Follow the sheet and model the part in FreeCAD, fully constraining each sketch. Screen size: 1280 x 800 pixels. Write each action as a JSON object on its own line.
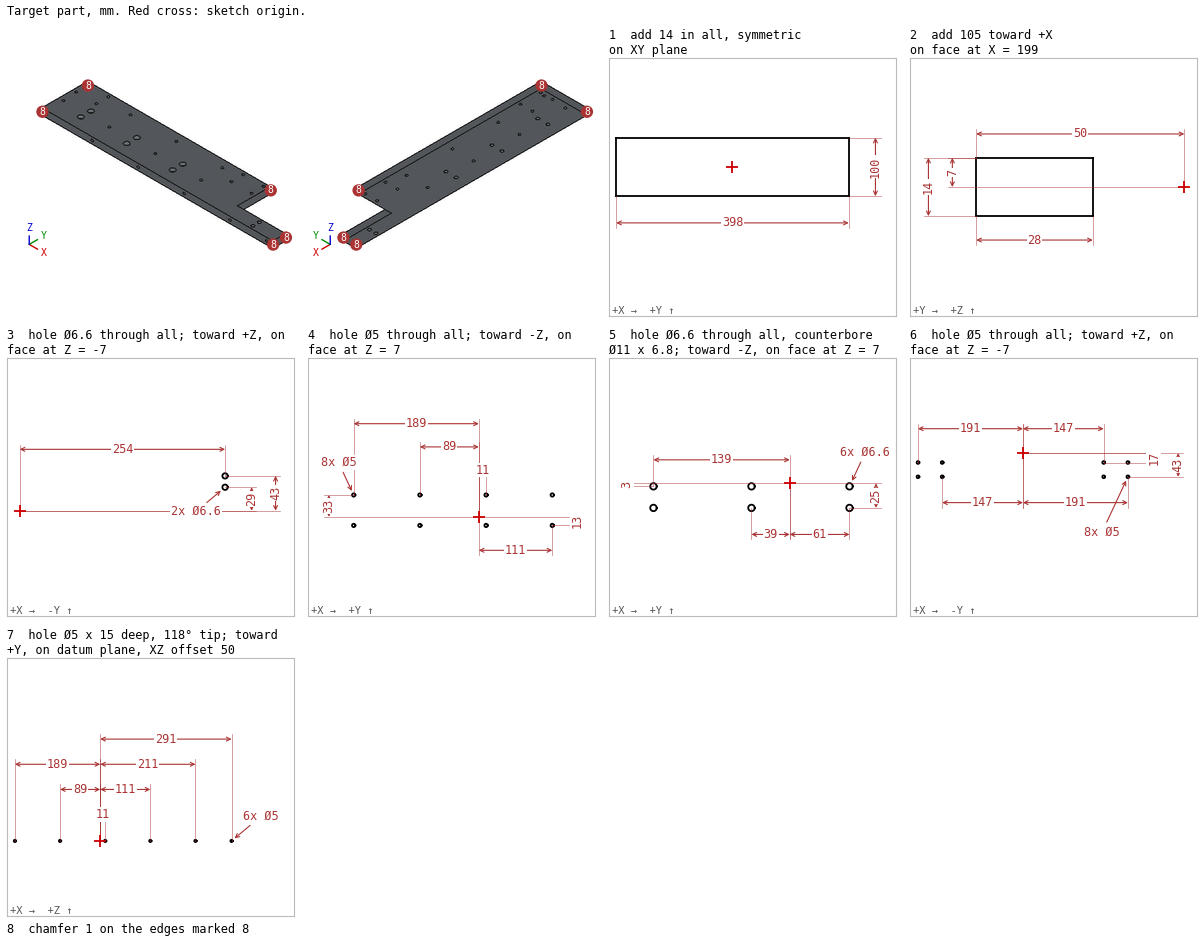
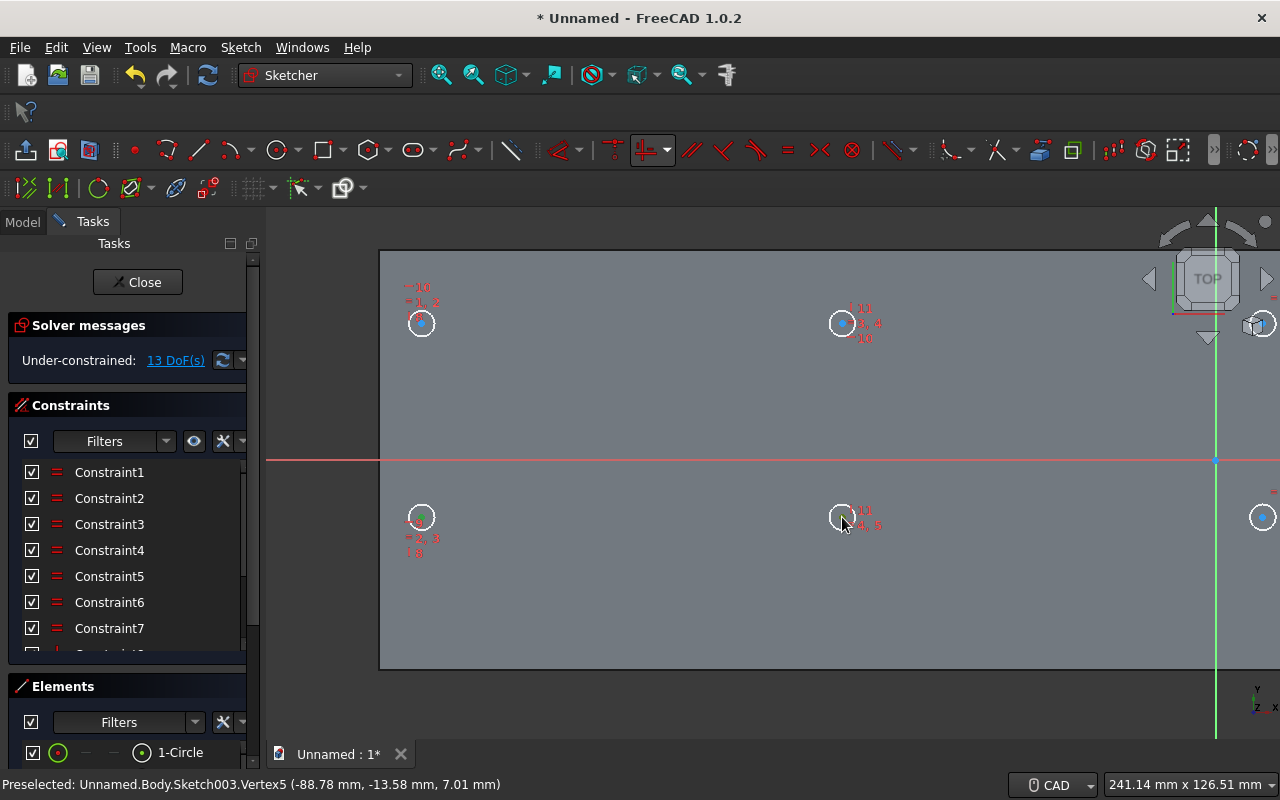
{"action": "left_click", "coordinate": [670, 150]}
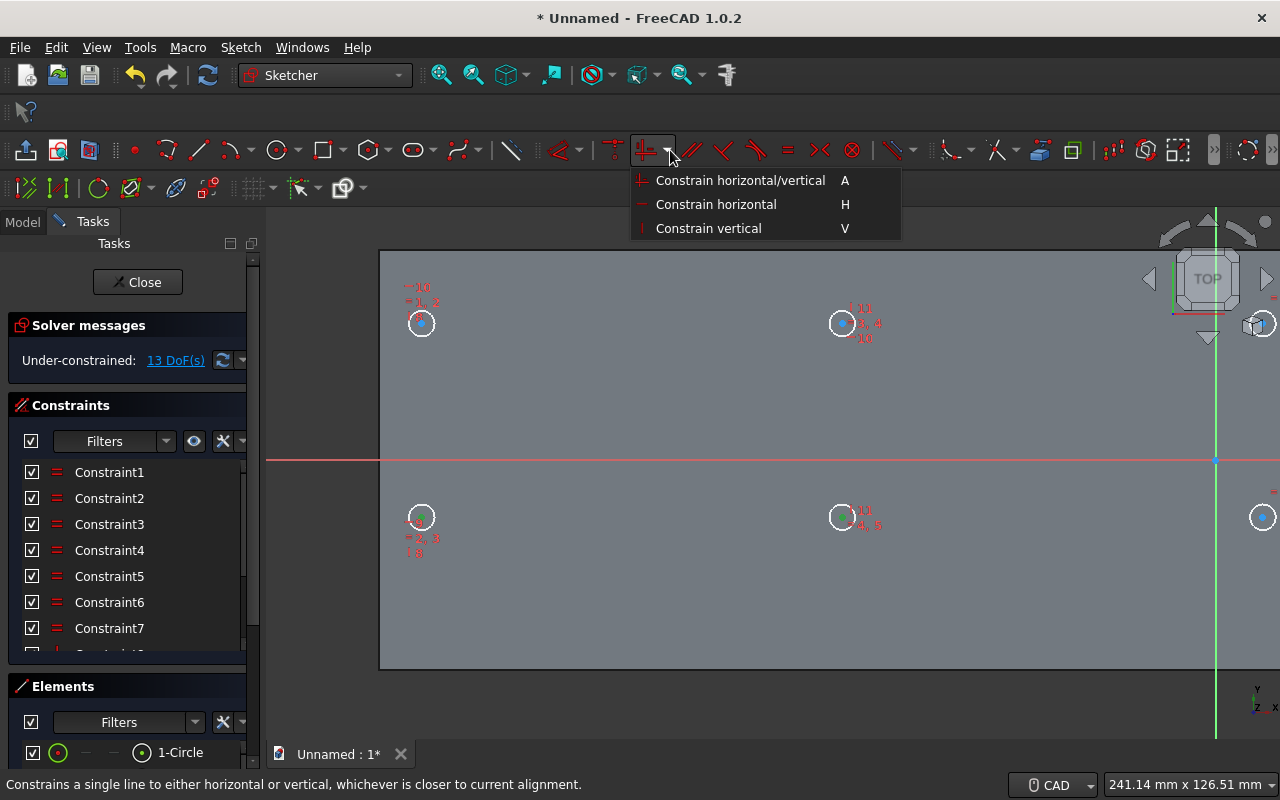
{"action": "left_click", "coordinate": [766, 204]}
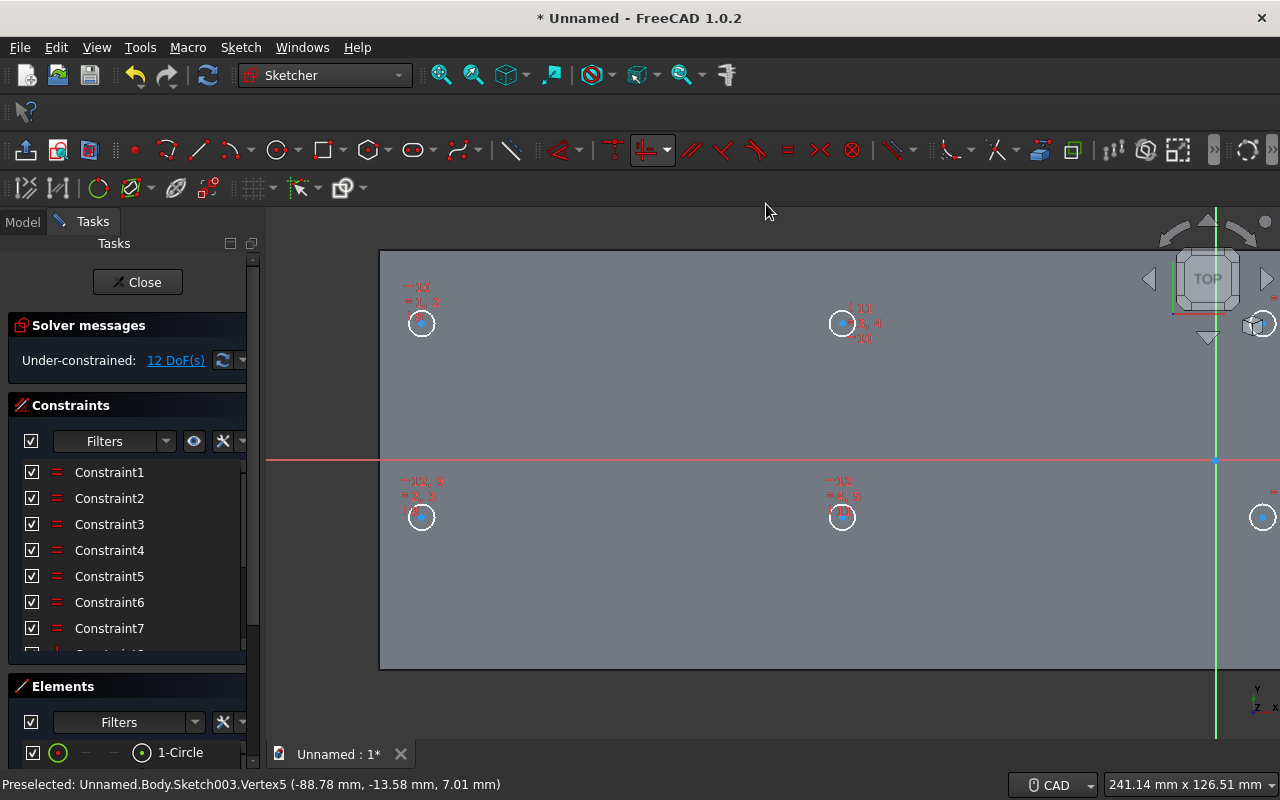
{"action": "left_click", "coordinate": [842, 324]}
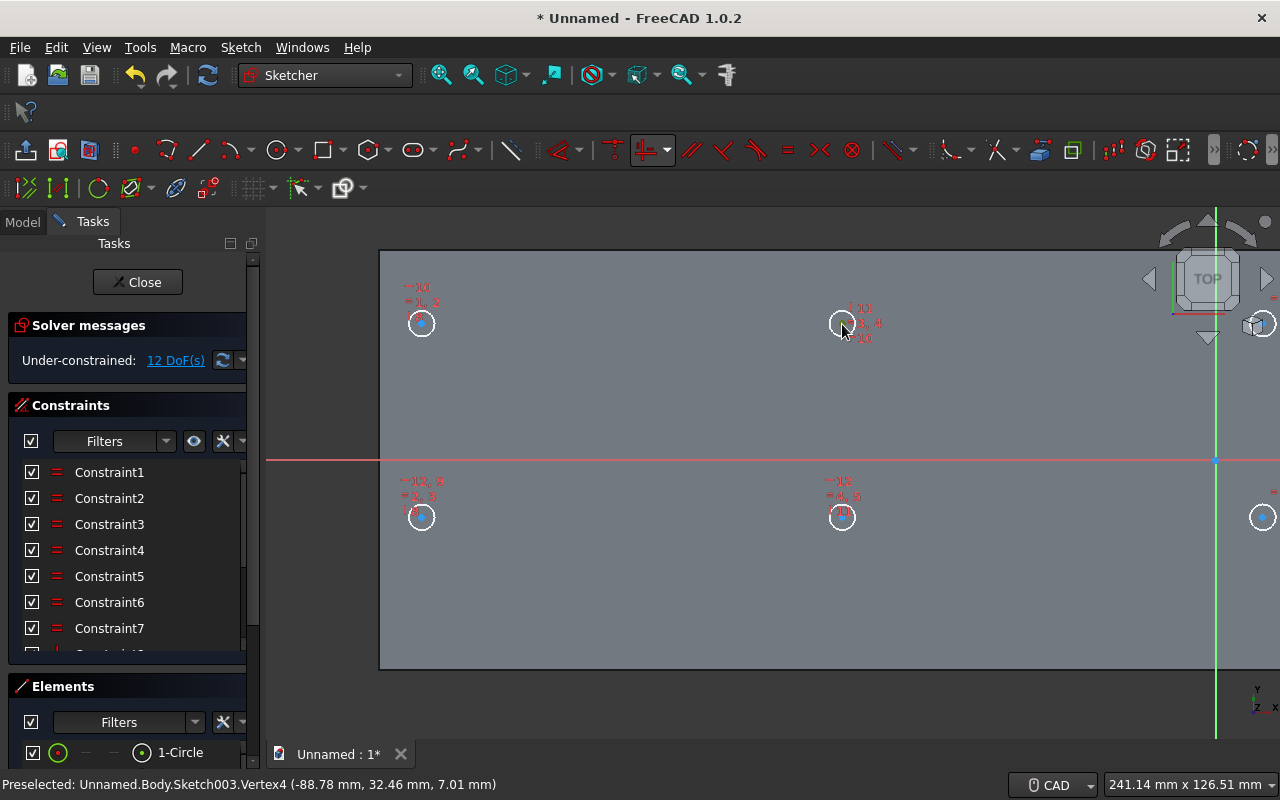
{"action": "scroll", "coordinate": [421, 518], "scroll_direction": "down", "scroll_amount": 4}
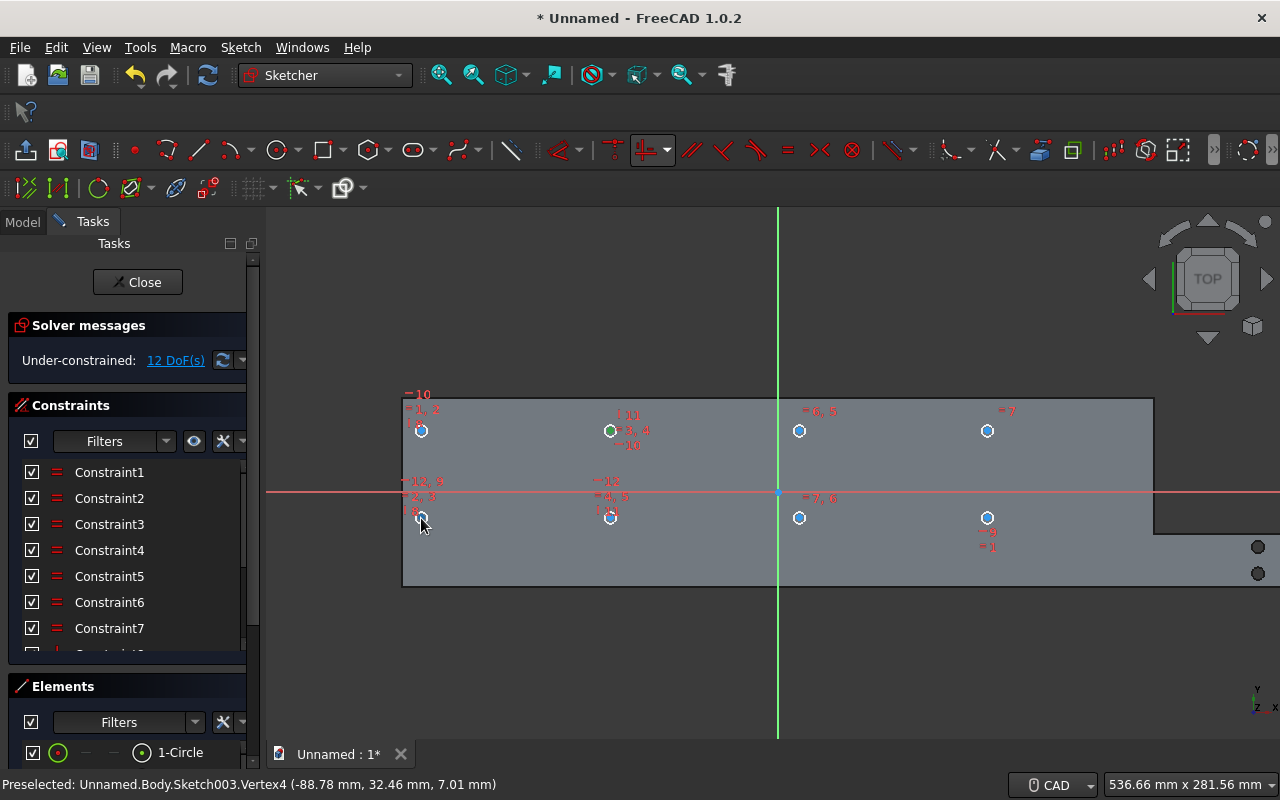
{"action": "left_click", "coordinate": [799, 431]}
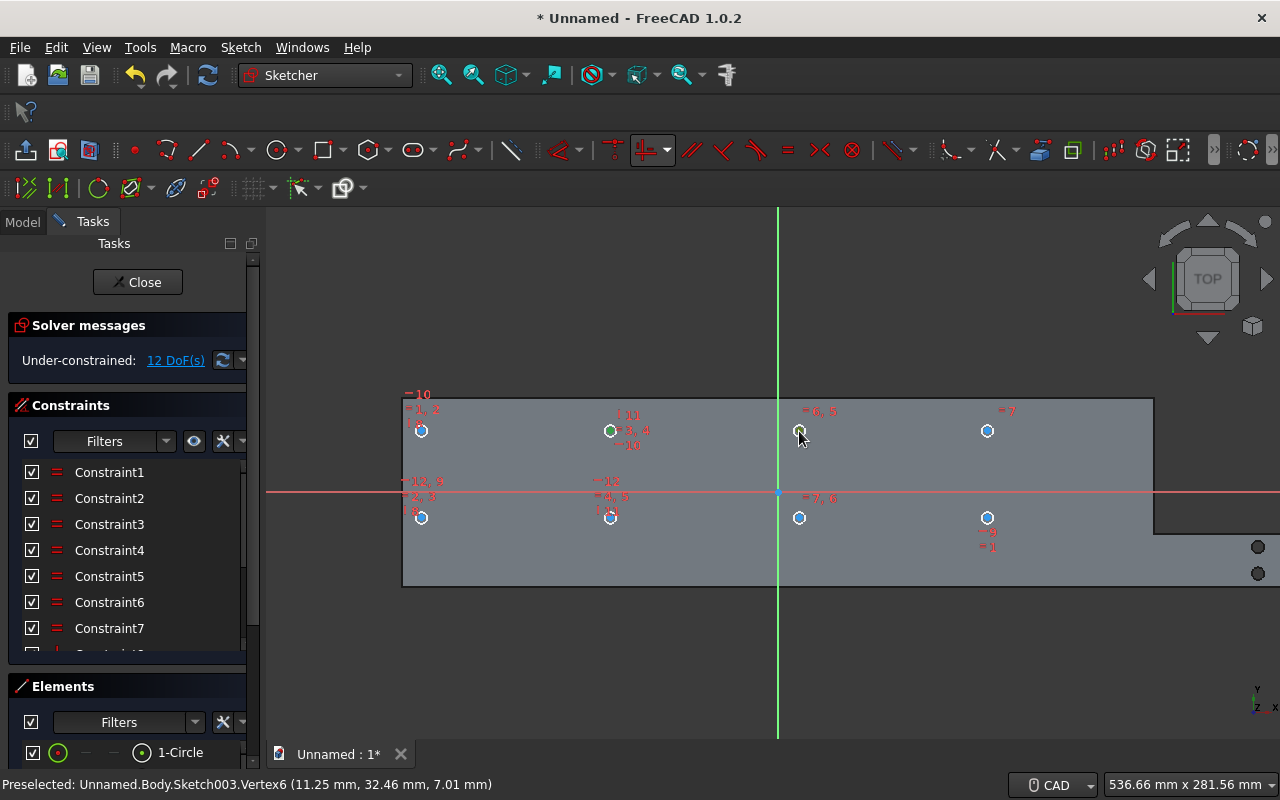
{"action": "key", "text": "h"}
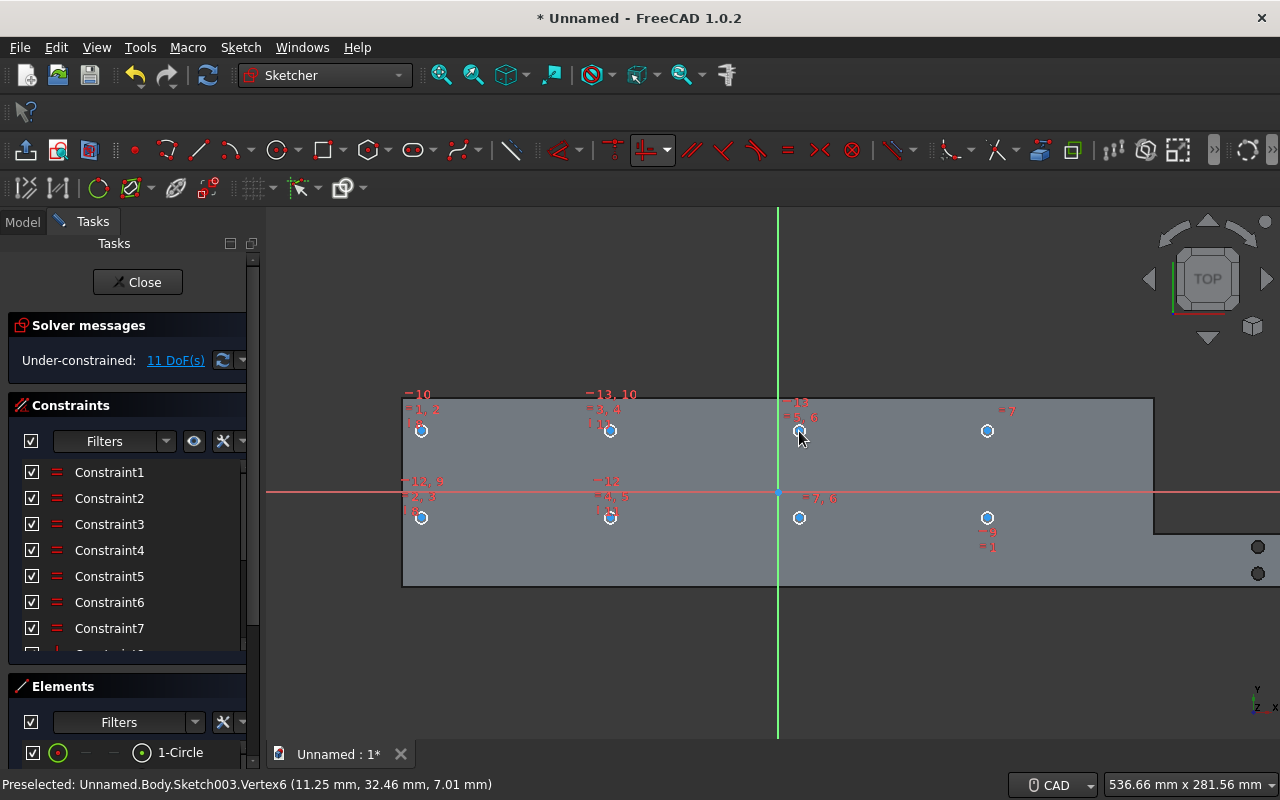
{"action": "left_click", "coordinate": [799, 431]}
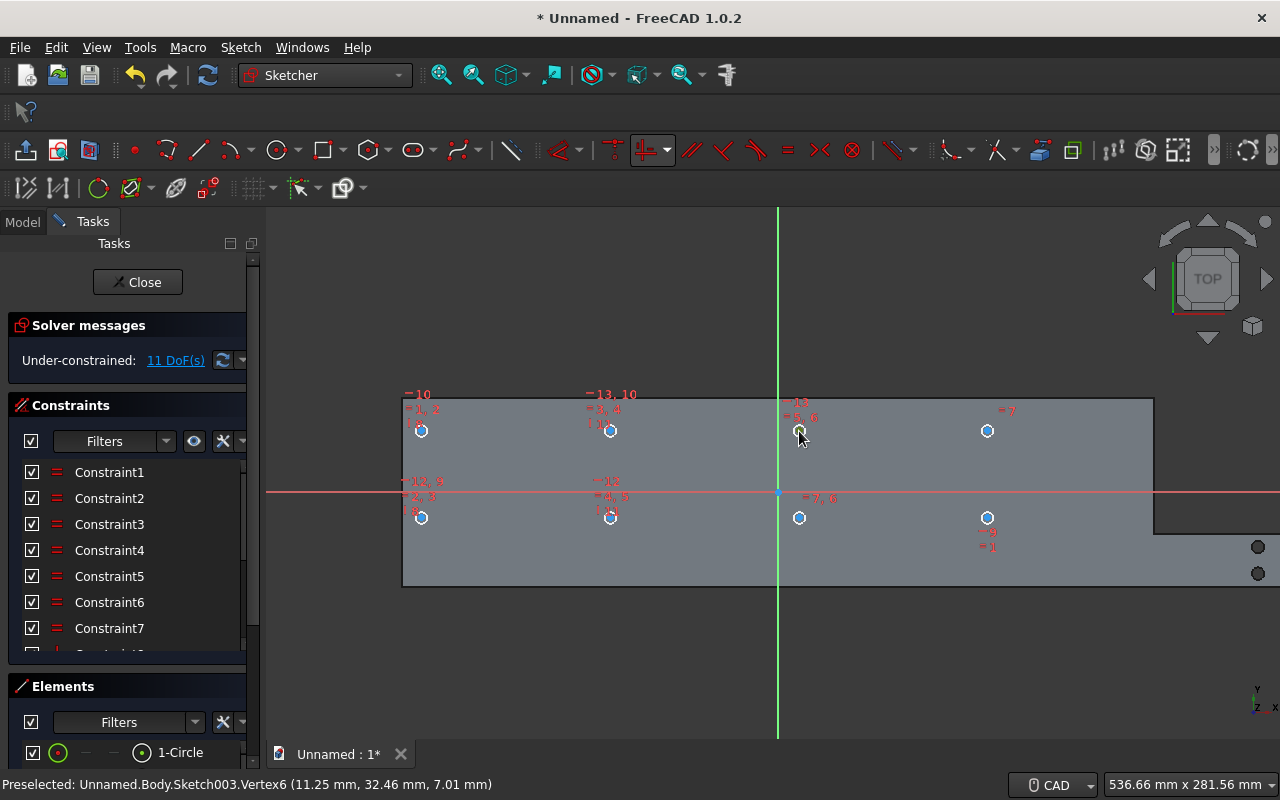
{"action": "left_click", "coordinate": [799, 518]}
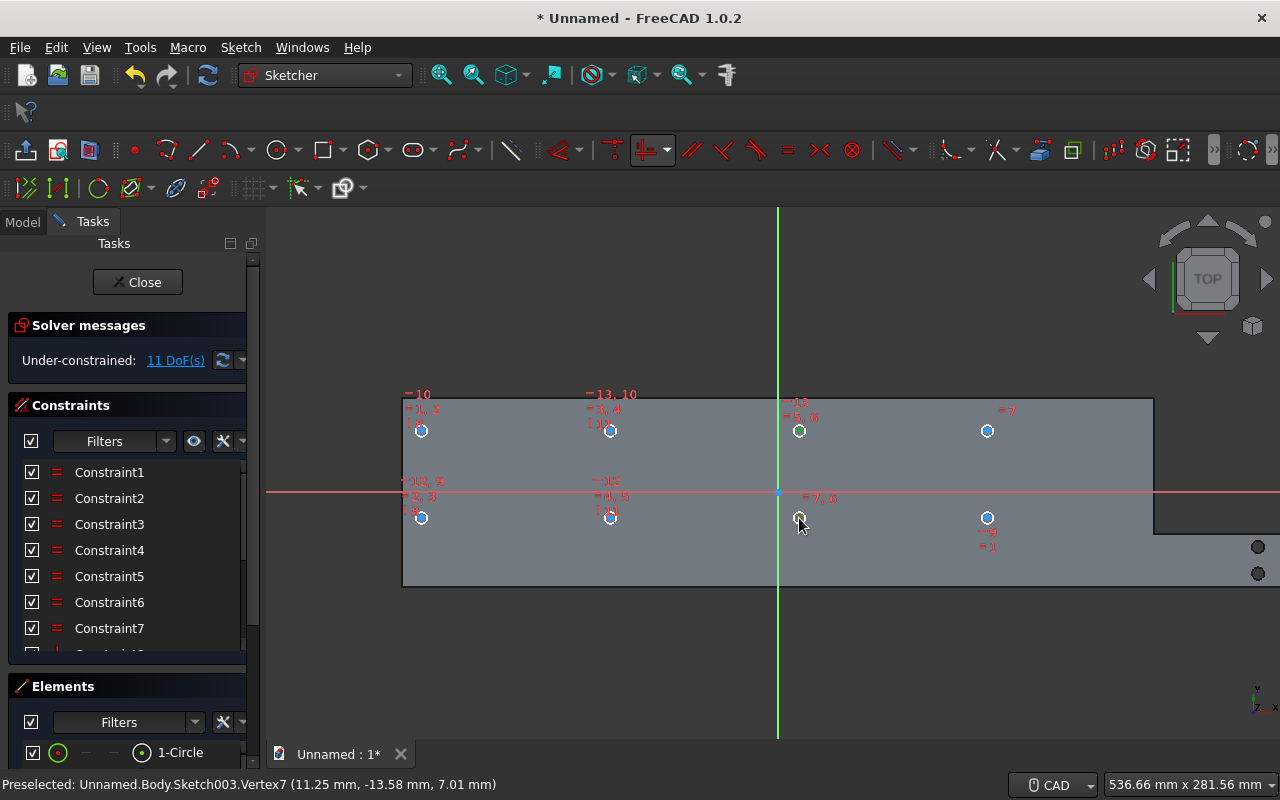
{"action": "key", "text": "v"}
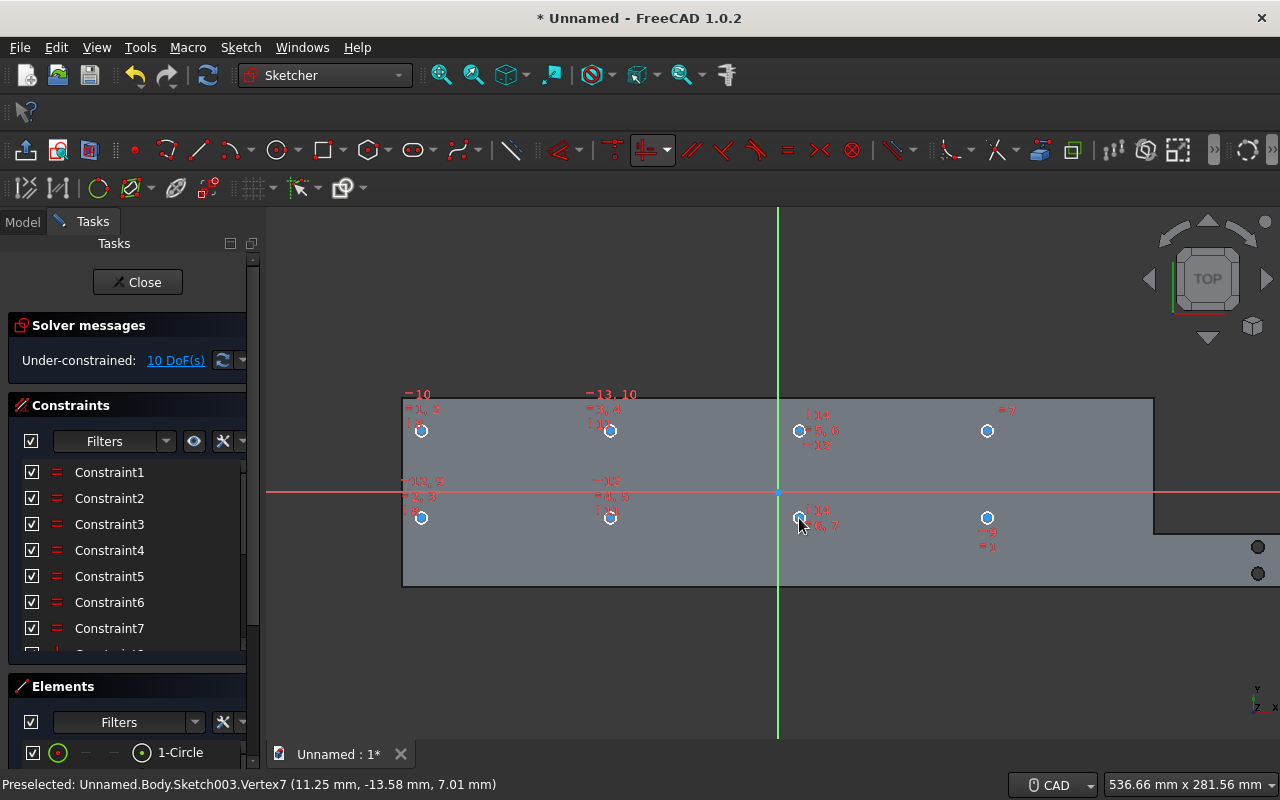
{"action": "left_click", "coordinate": [987, 518]}